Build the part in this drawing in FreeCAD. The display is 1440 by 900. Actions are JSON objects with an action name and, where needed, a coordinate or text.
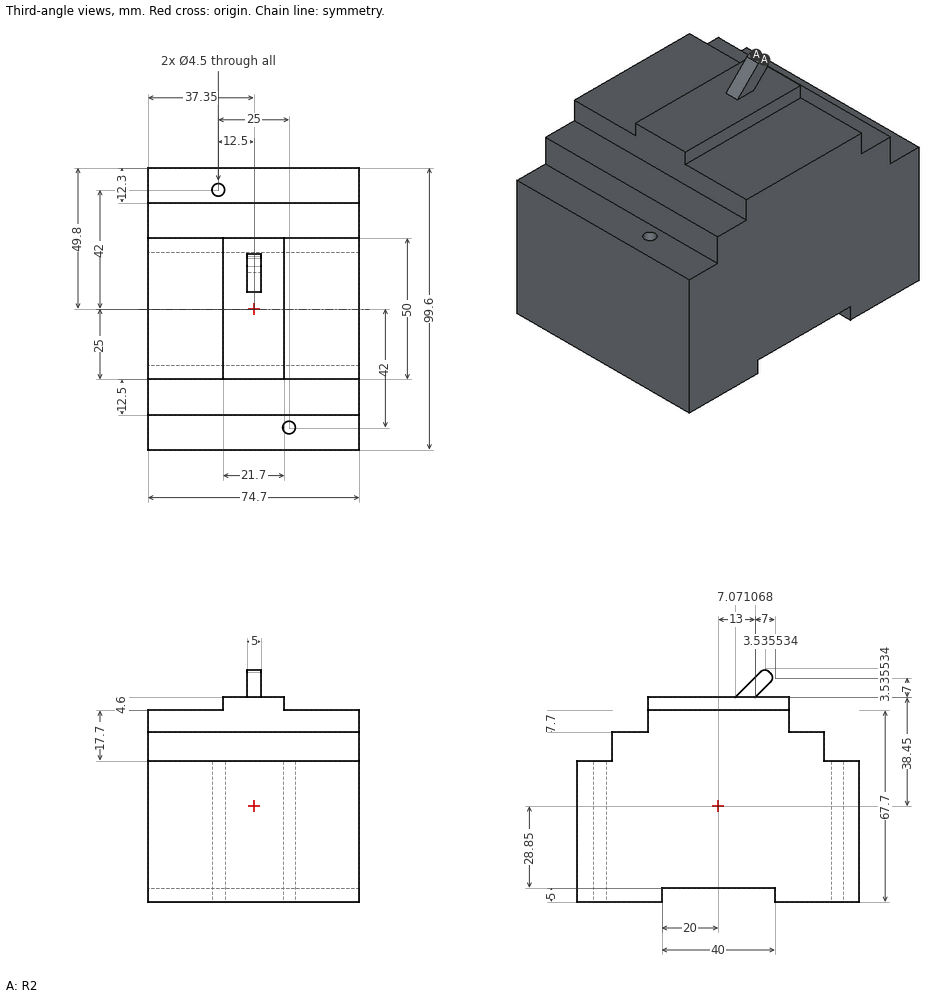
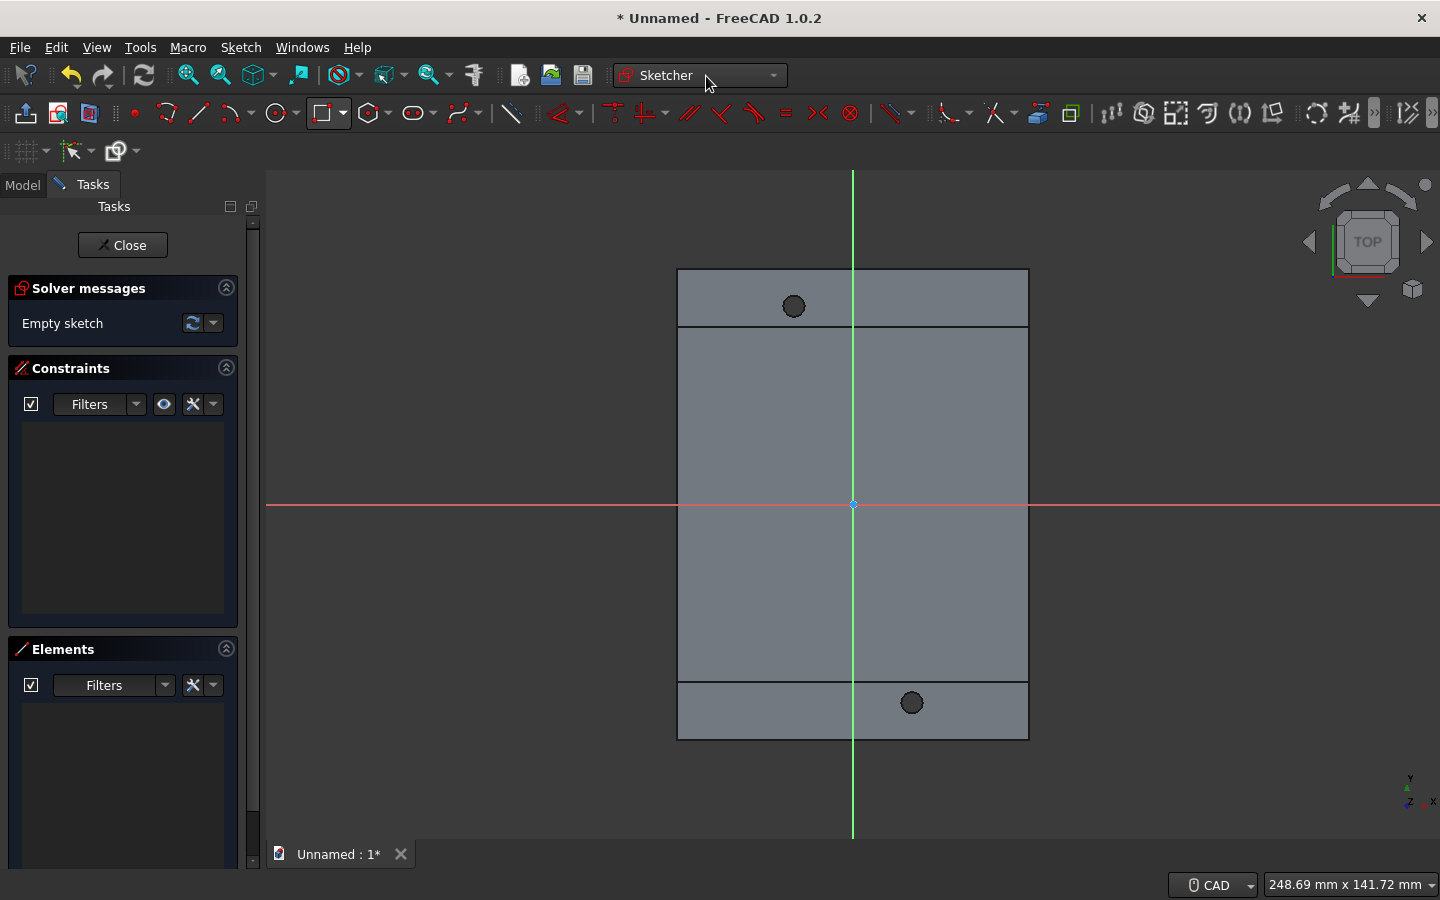
{"action": "left_click", "coordinate": [322, 114]}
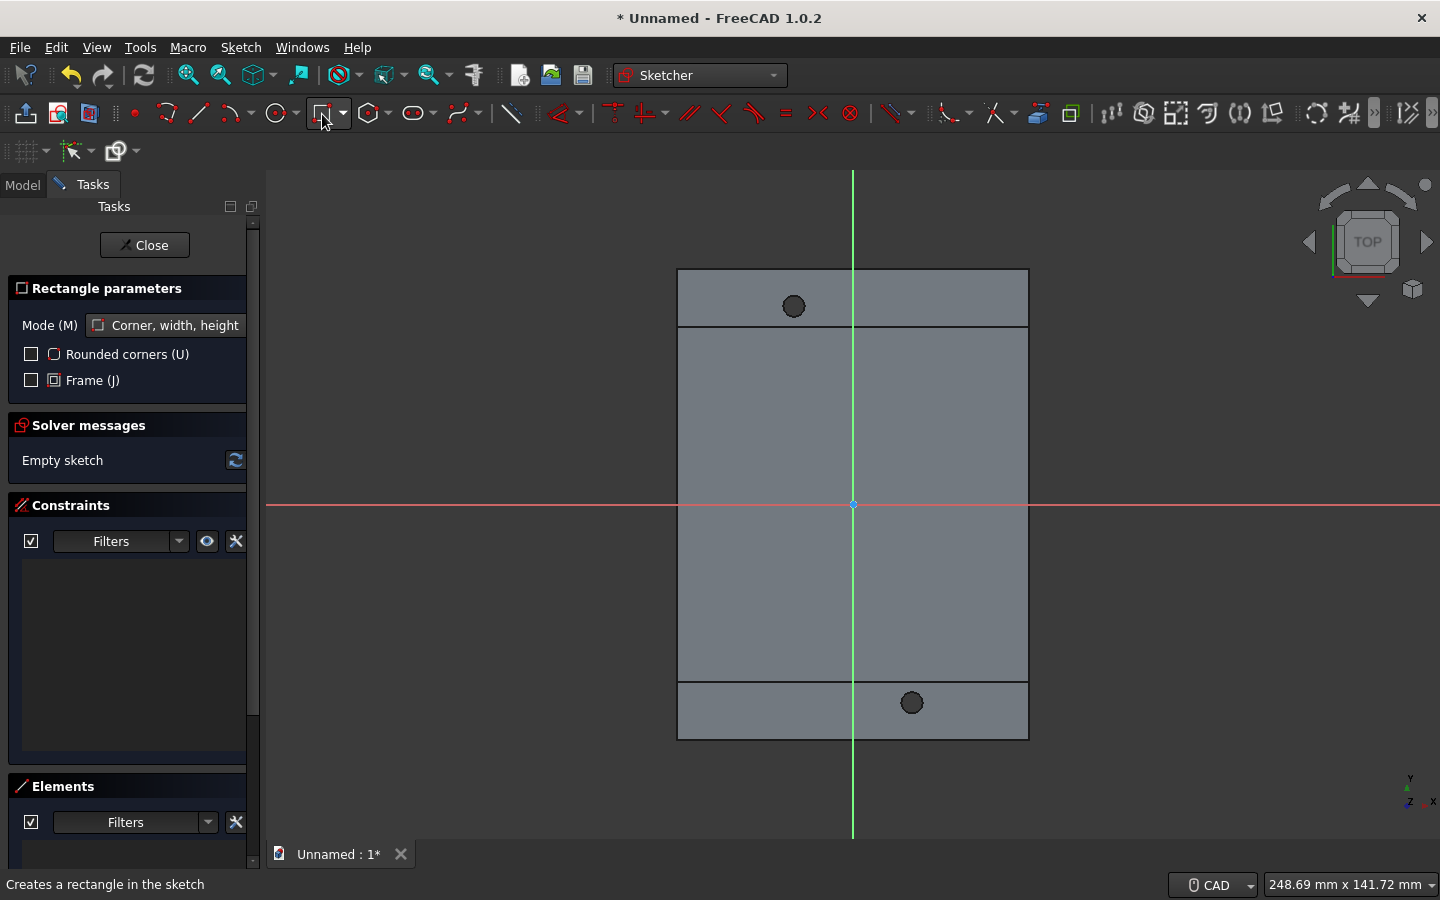
{"action": "left_click", "coordinate": [677, 623]}
{"action": "left_click", "coordinate": [1029, 682]}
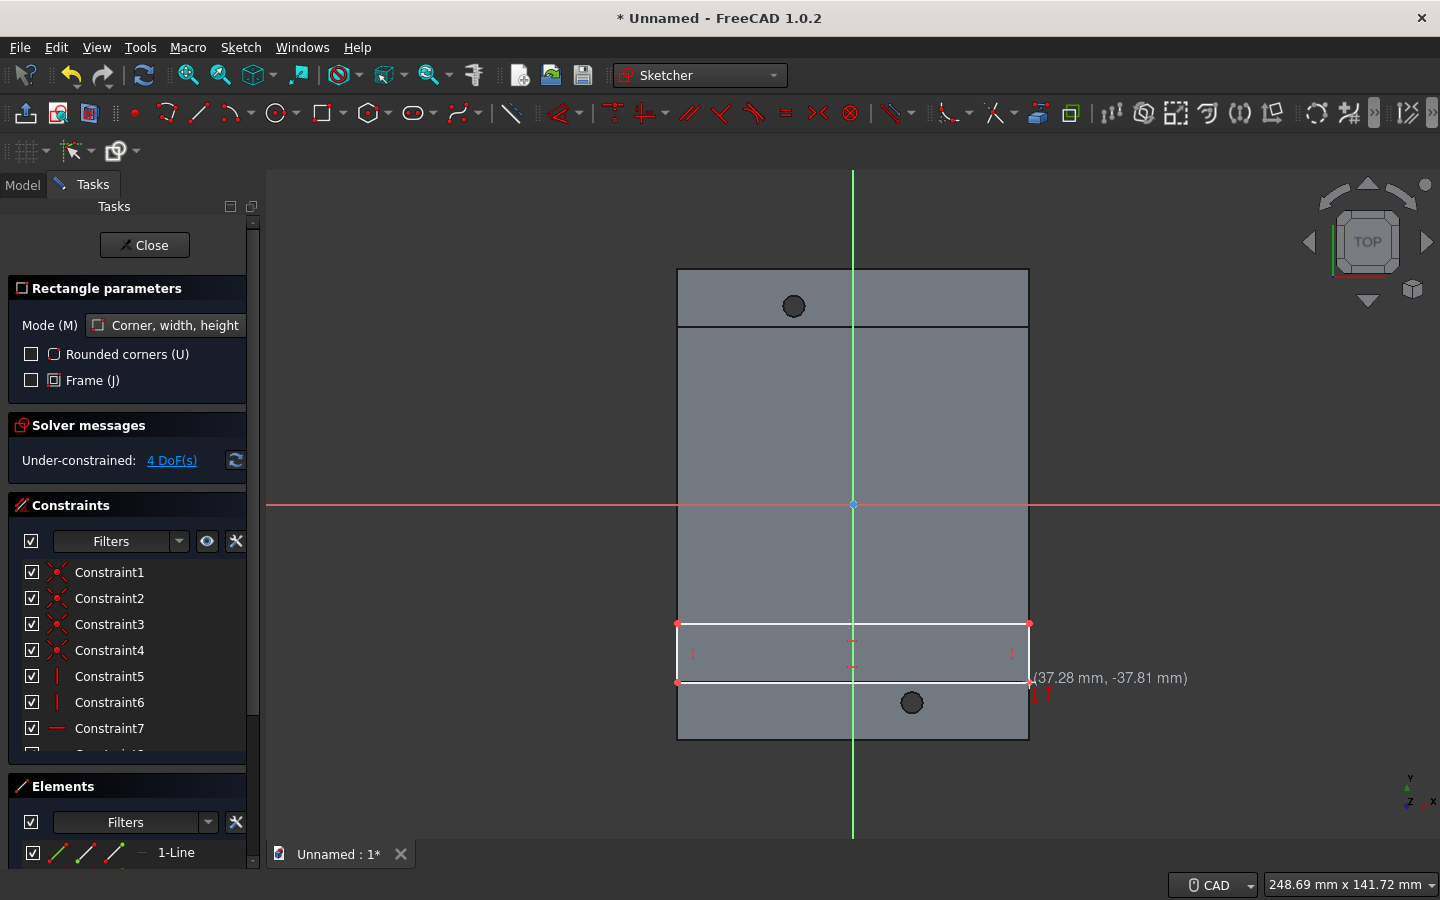
{"action": "left_click", "coordinate": [677, 327]}
{"action": "left_click", "coordinate": [1029, 386]}
{"action": "key", "text": "Escape"}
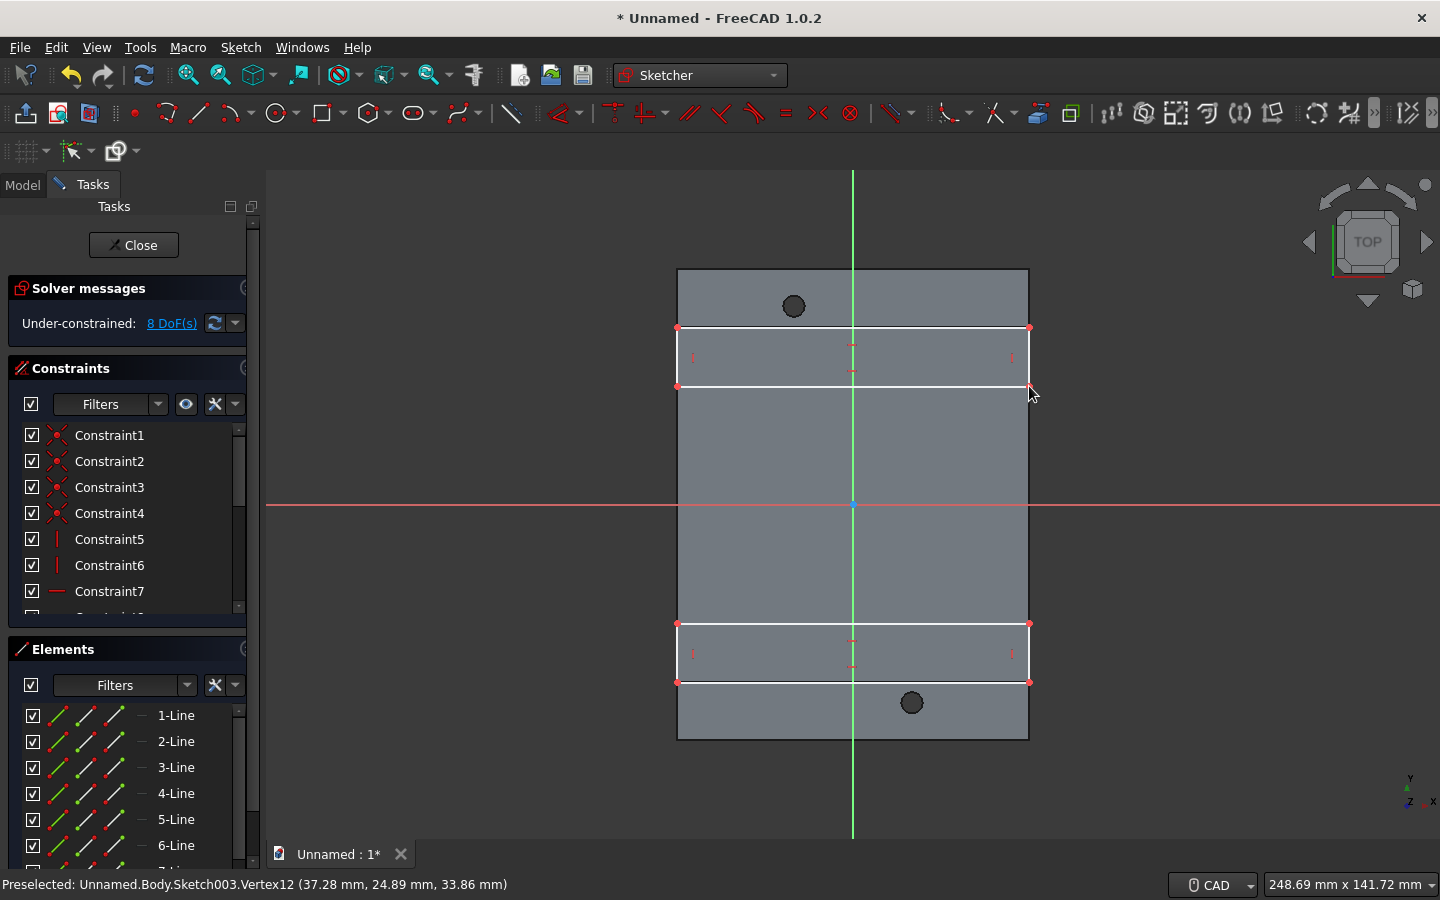
{"action": "left_click", "coordinate": [677, 683]}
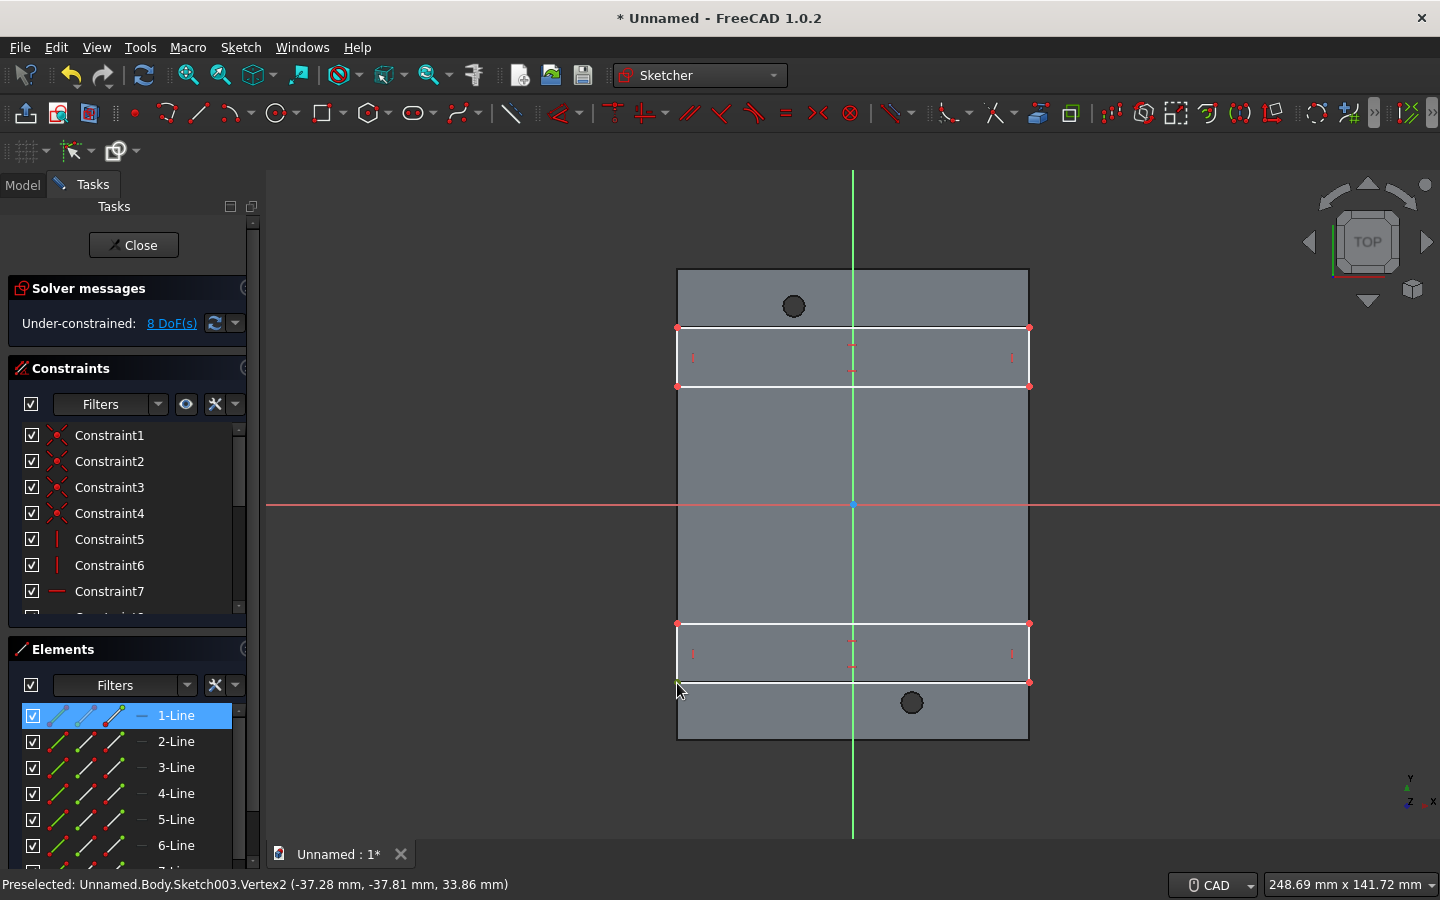
{"action": "left_click", "coordinate": [677, 328]}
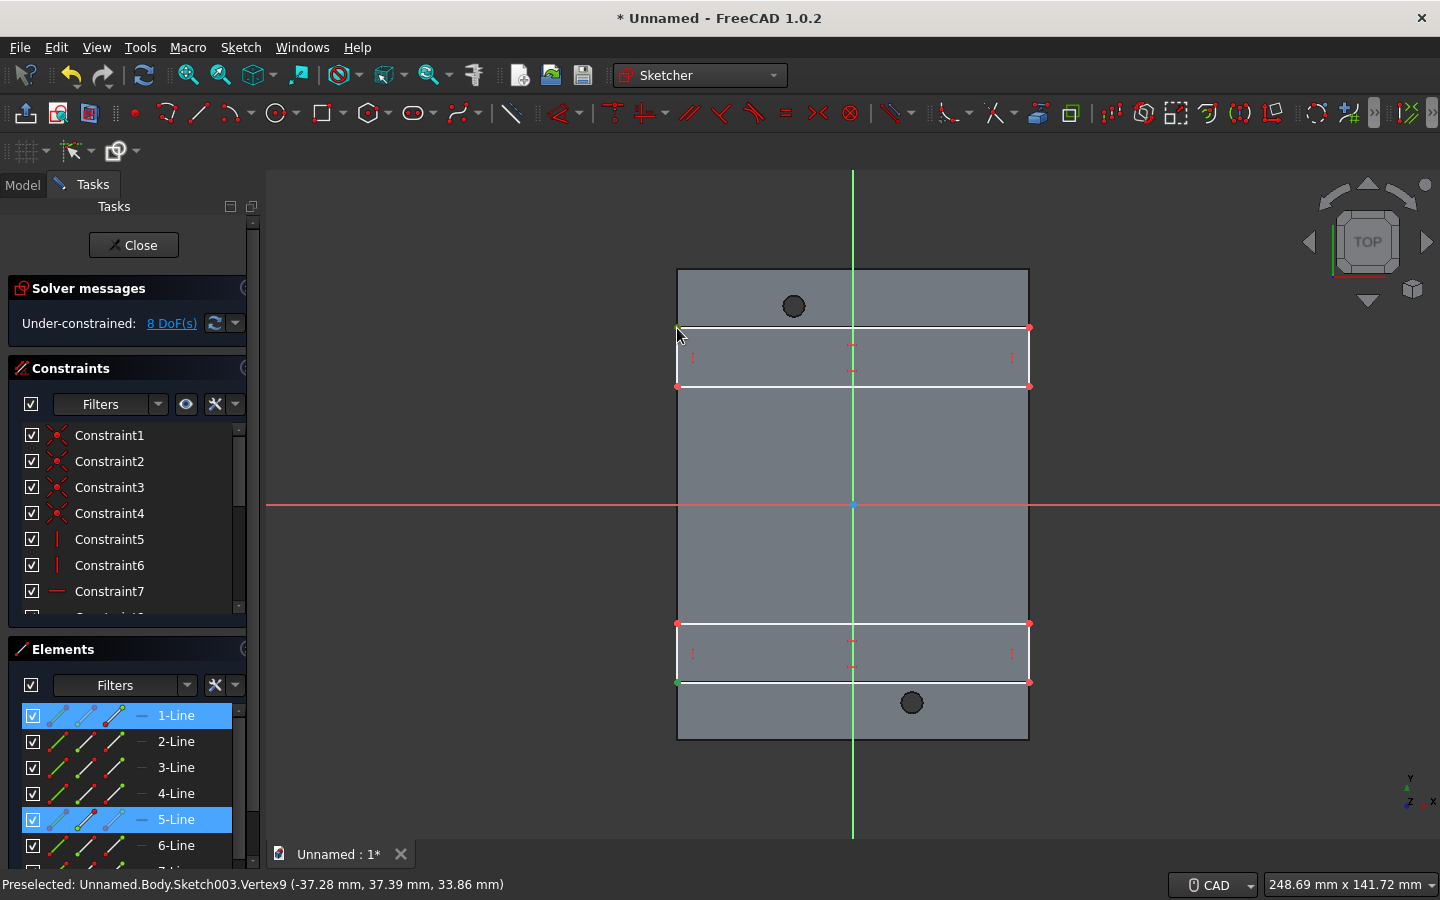
{"action": "left_click", "coordinate": [364, 504]}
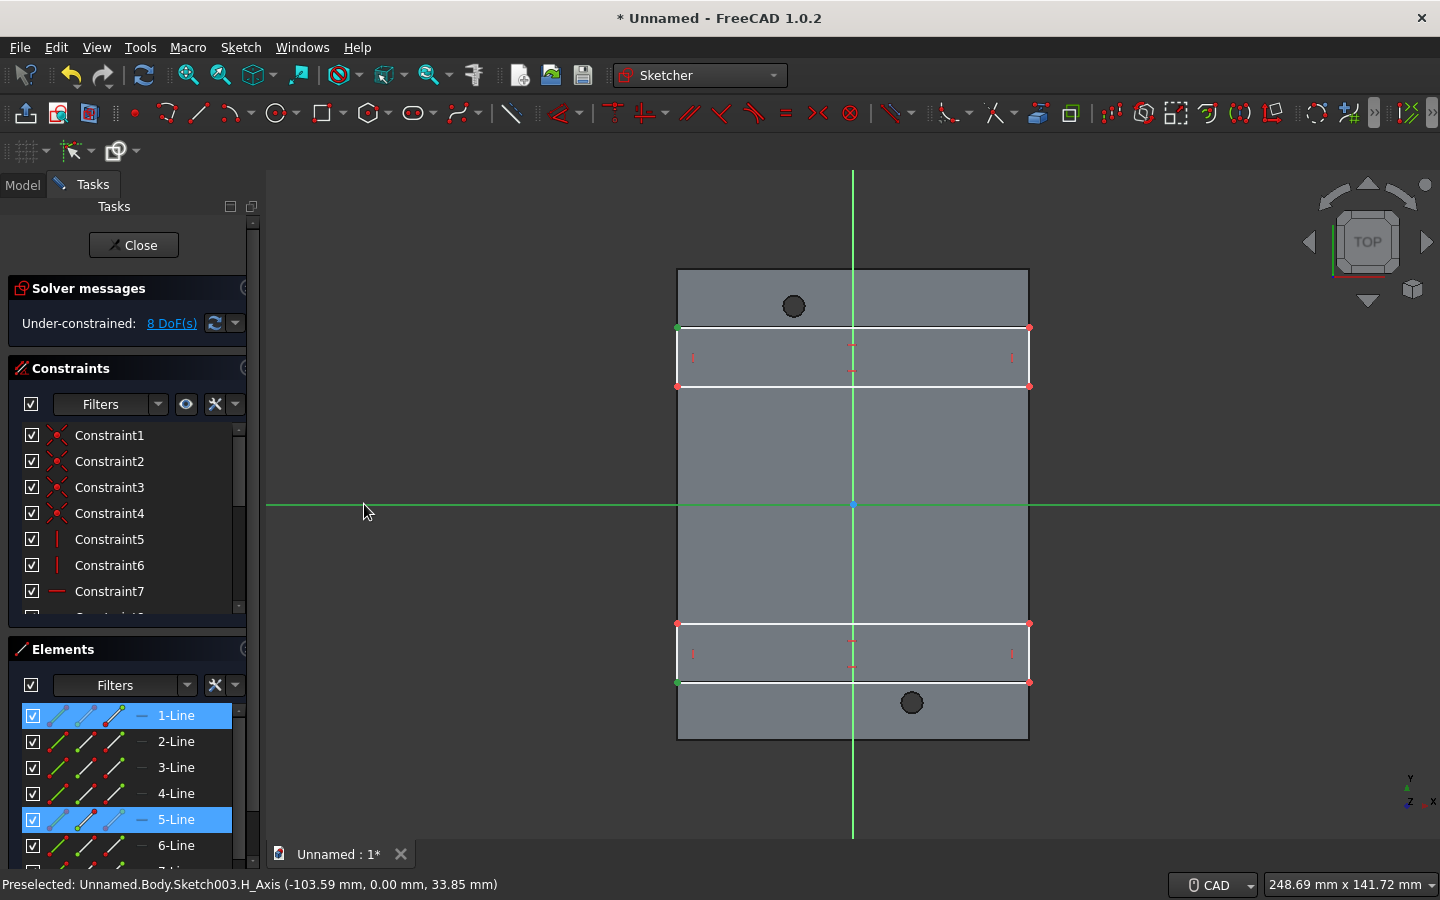
{"action": "left_click", "coordinate": [818, 114]}